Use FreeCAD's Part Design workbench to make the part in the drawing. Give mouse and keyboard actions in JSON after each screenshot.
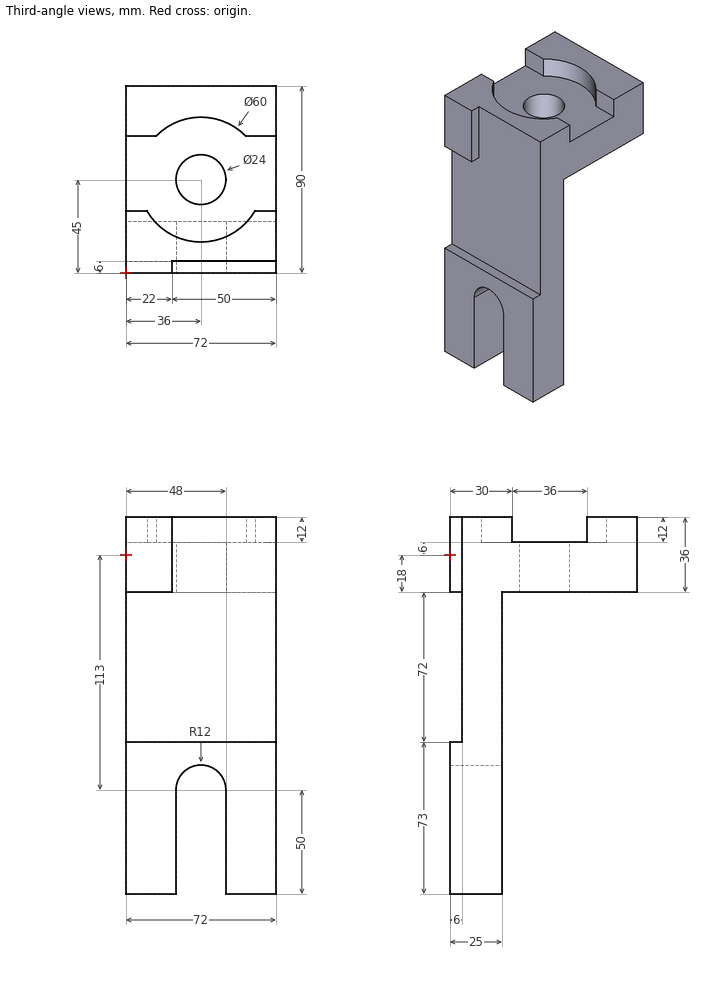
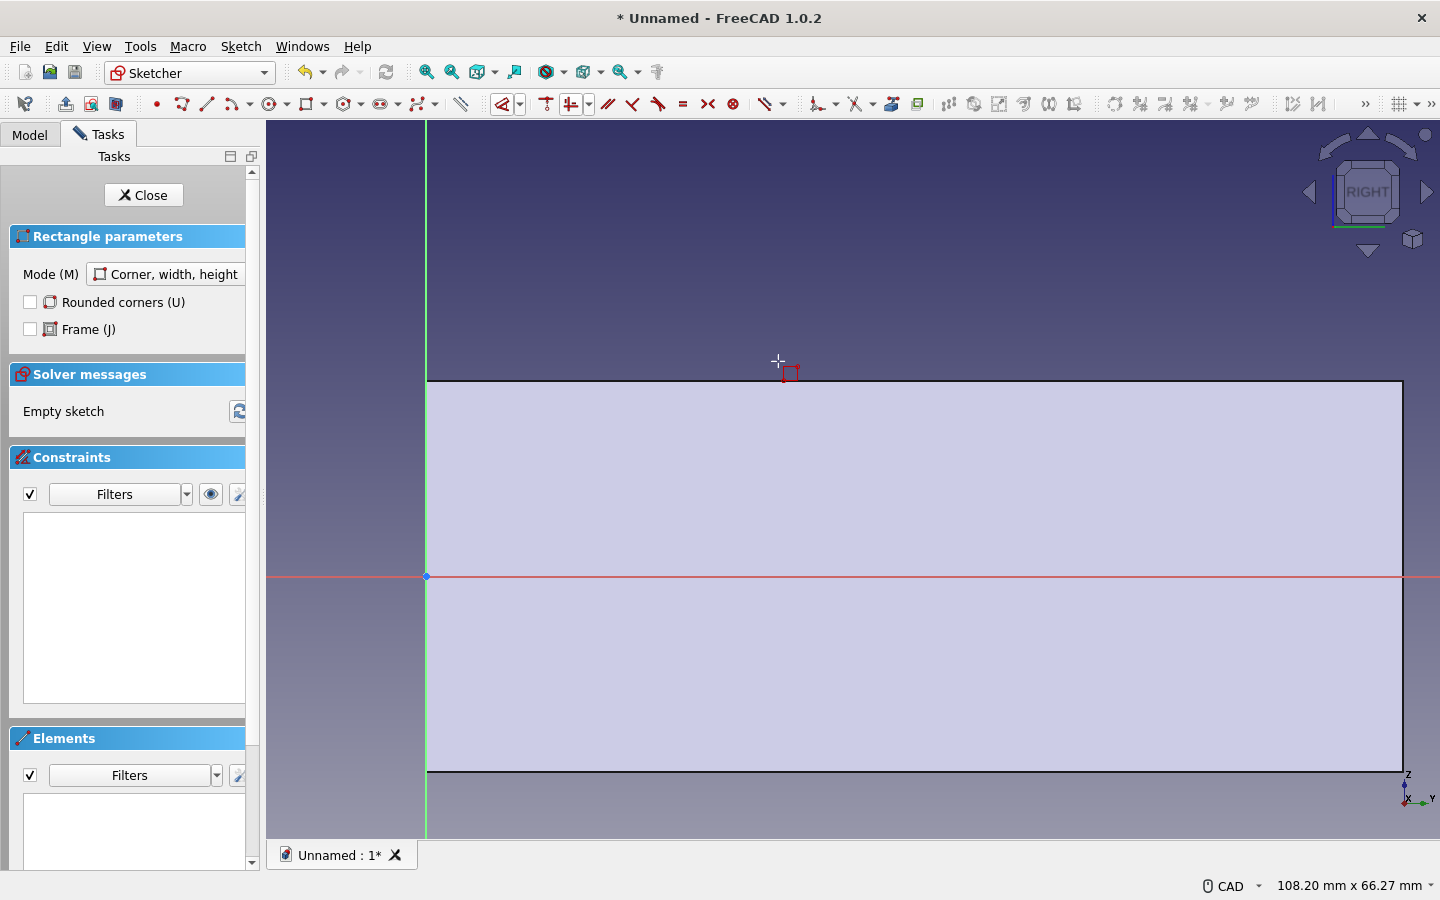
{"action": "left_click", "coordinate": [752, 381]}
{"action": "mouse_move", "coordinate": [1142, 512]}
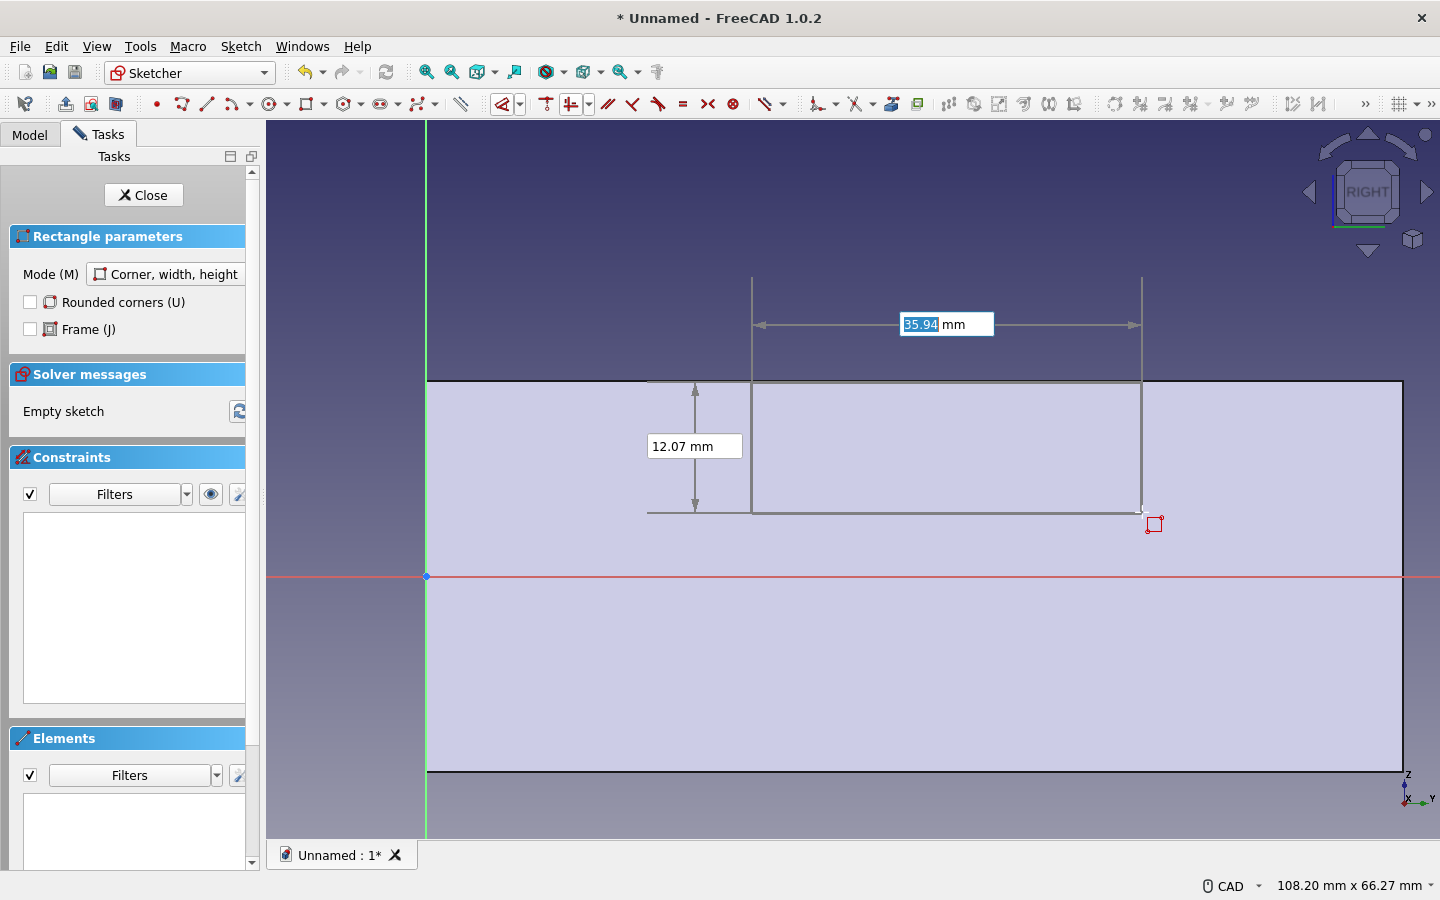
{"action": "type", "text": "36"}
{"action": "key", "text": "Tab"}
{"action": "type", "text": "12"}
{"action": "key", "text": "Return"}
{"action": "key", "text": "Escape"}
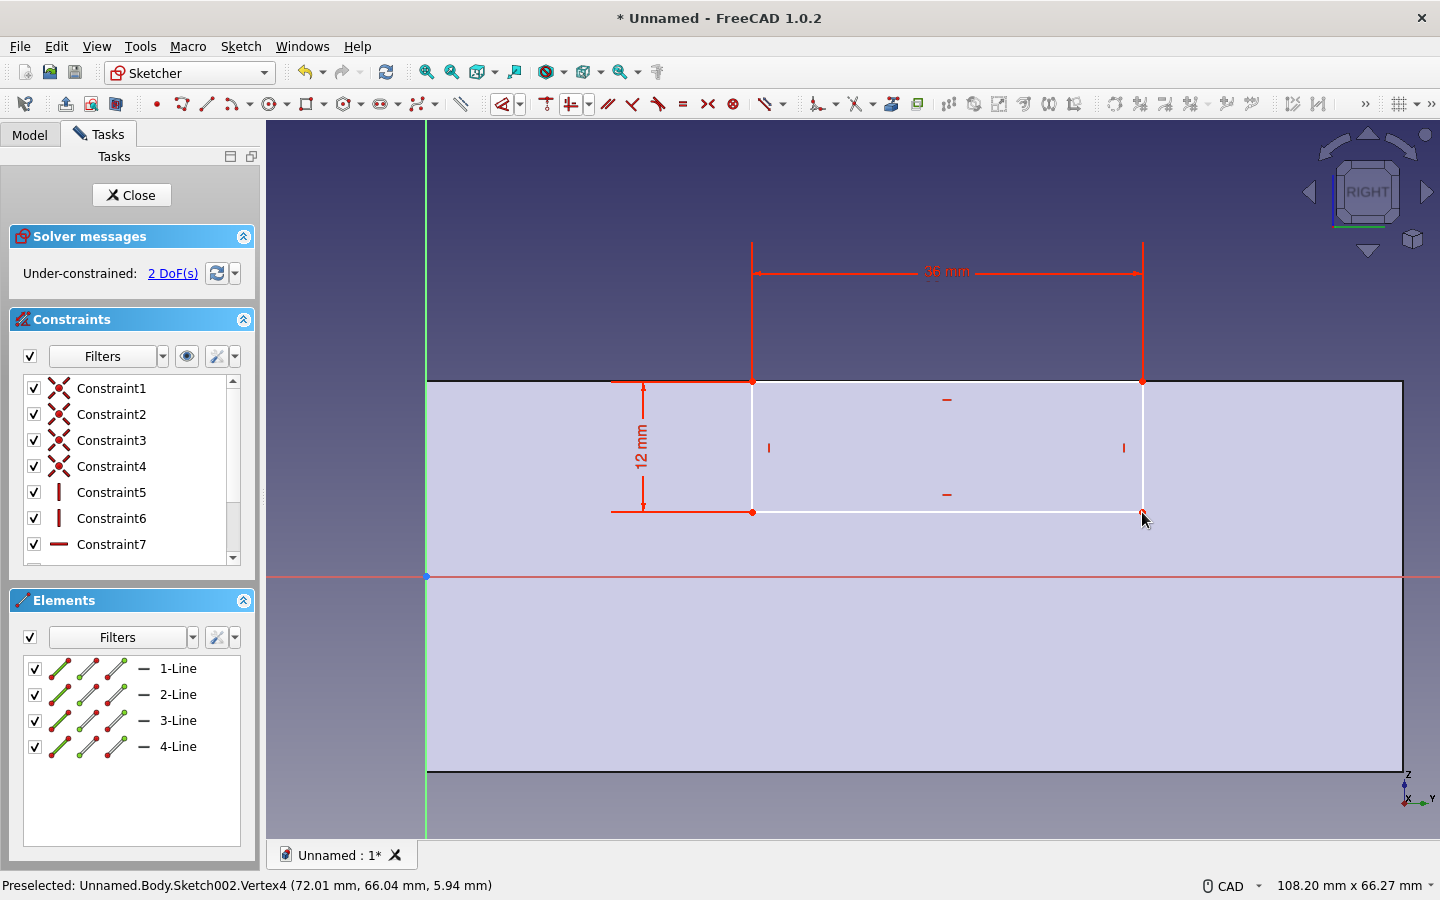
{"action": "key", "text": "d"}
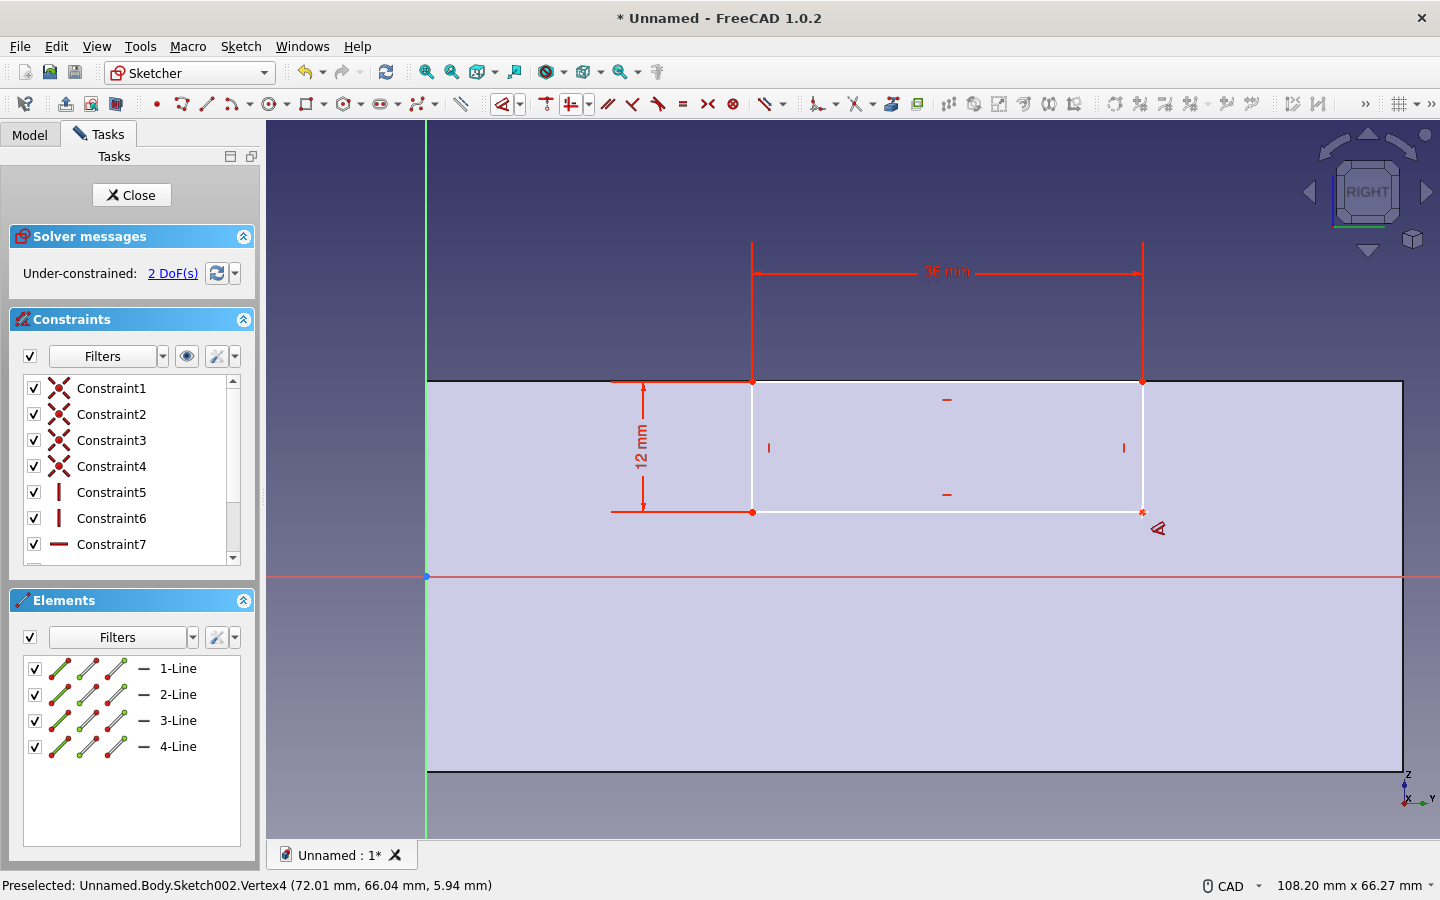
{"action": "left_click", "coordinate": [752, 512]}
{"action": "left_click", "coordinate": [392, 544]}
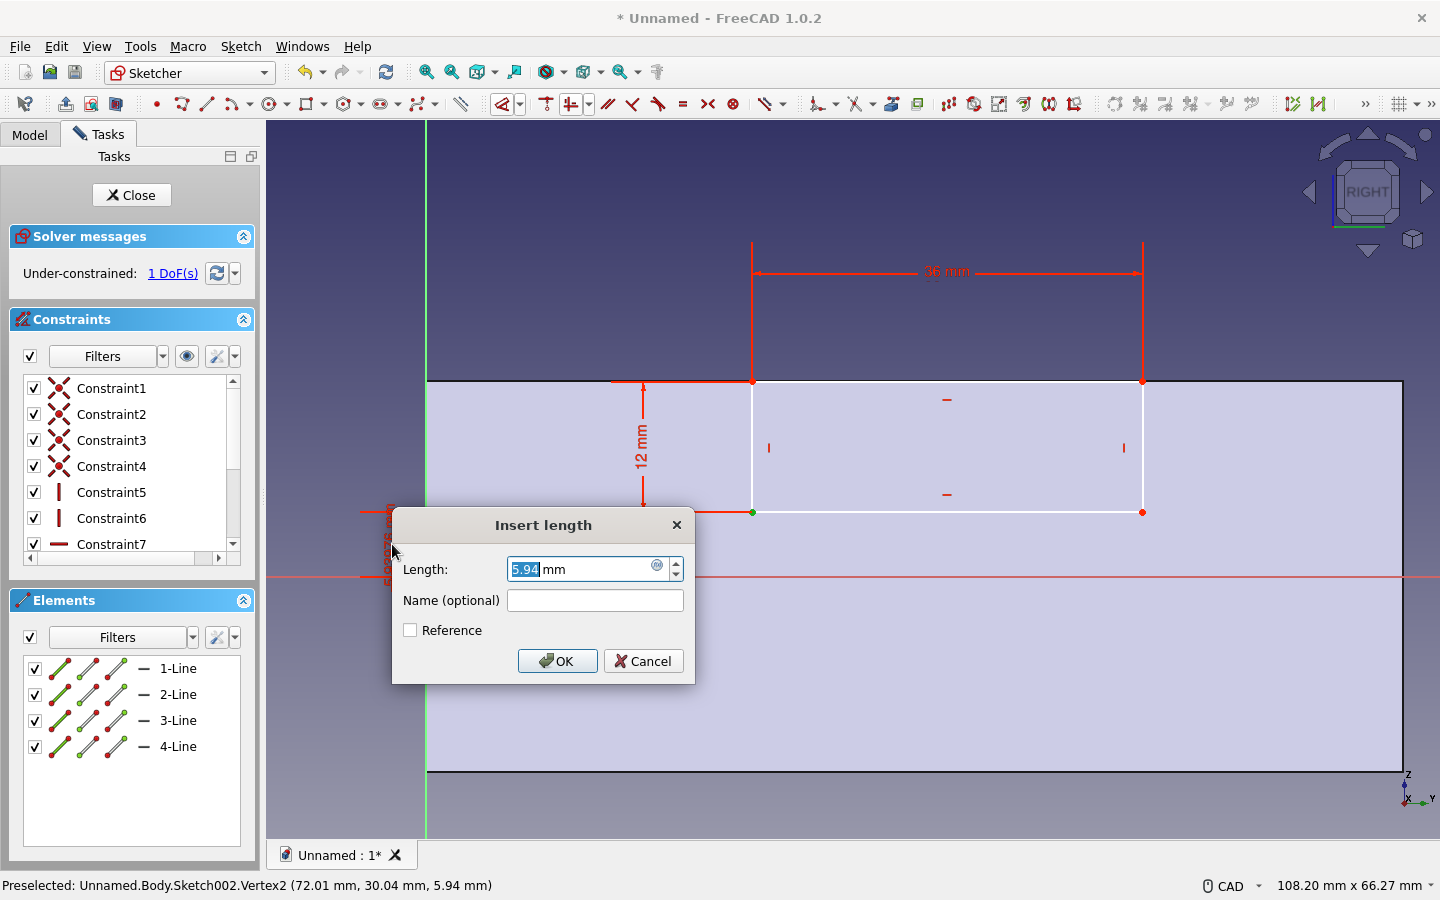
{"action": "type", "text": "6"}
{"action": "key", "text": "Return"}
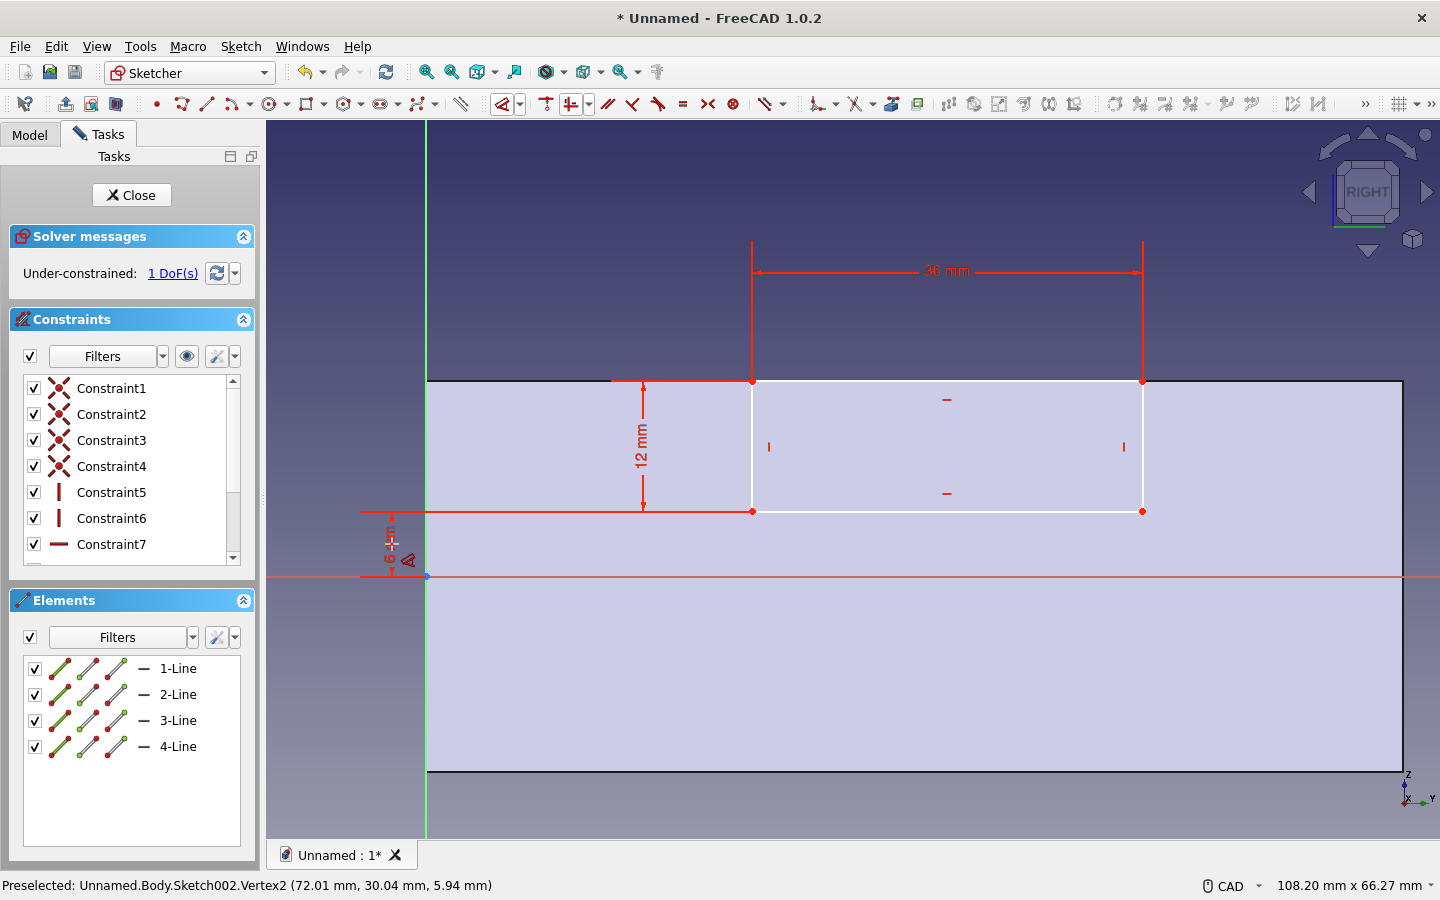
{"action": "left_click", "coordinate": [752, 381]}
{"action": "left_click", "coordinate": [589, 611]}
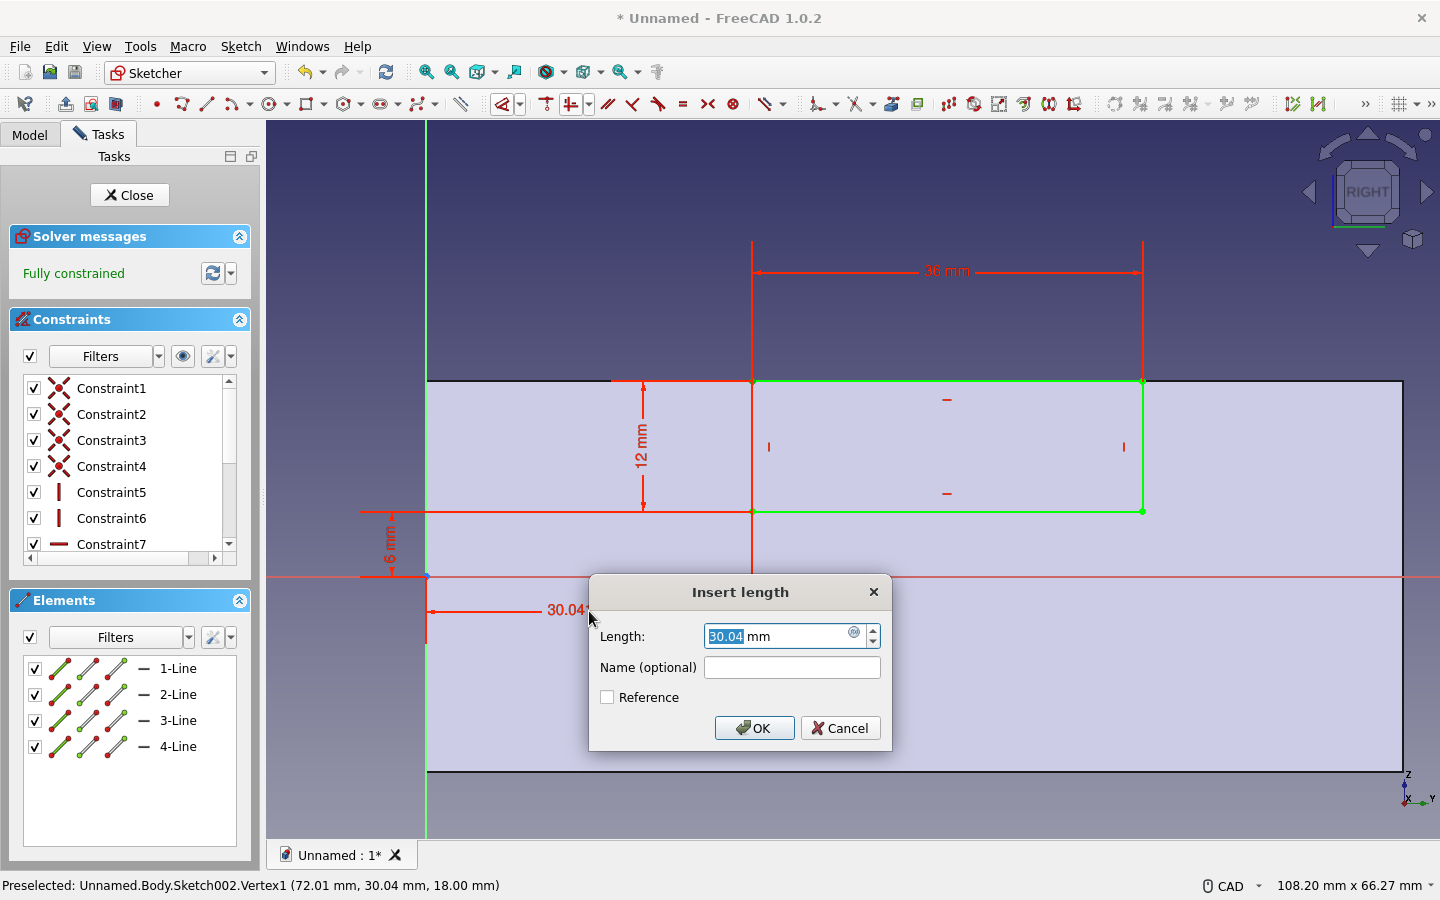
{"action": "type", "text": "30"}
{"action": "key", "text": "Return"}
{"action": "key", "text": "Escape"}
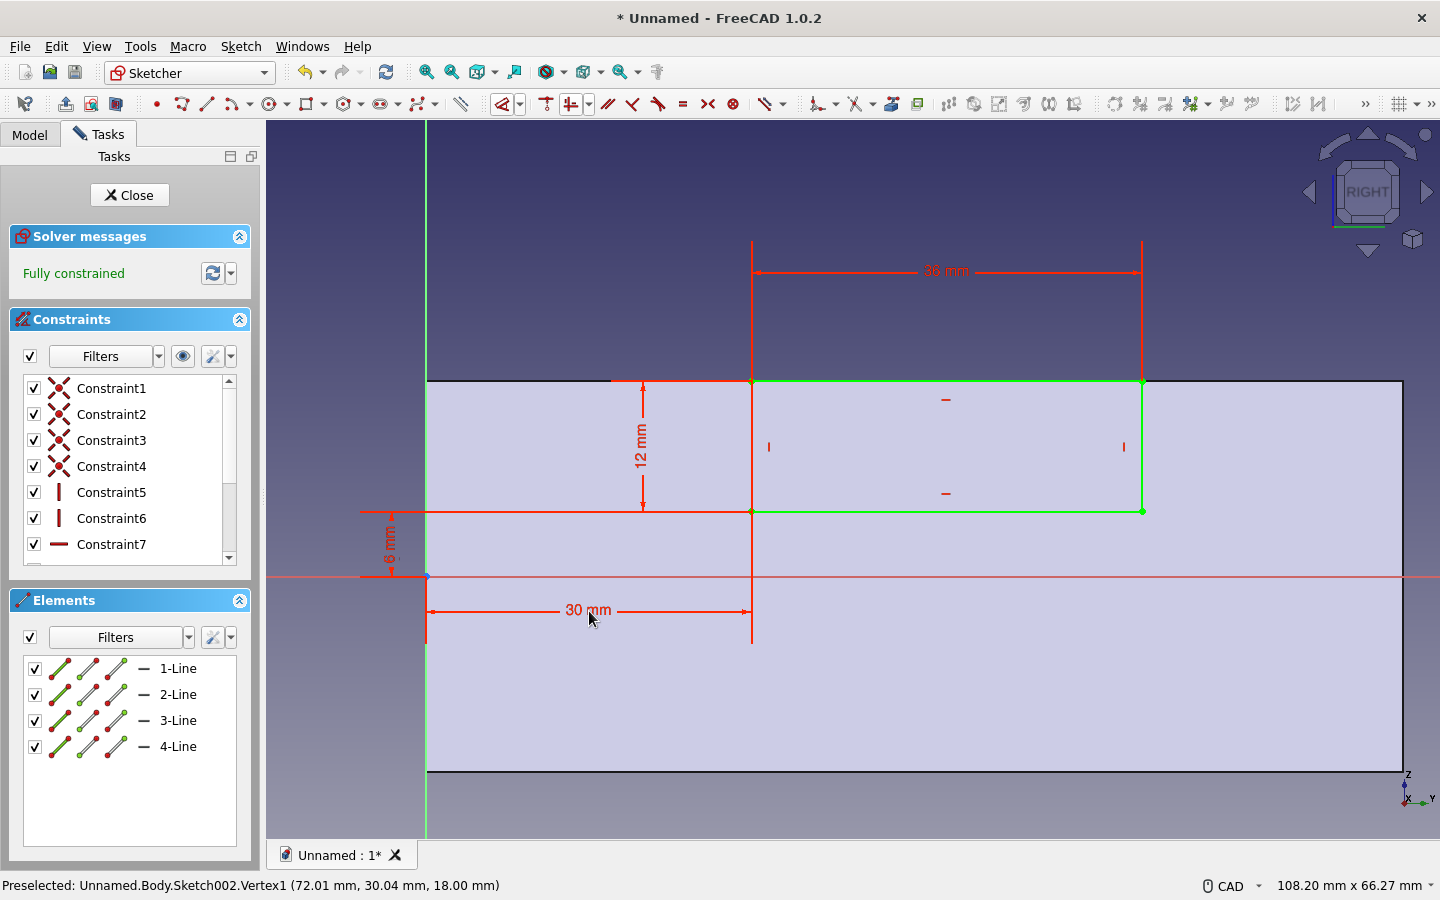
{"action": "left_click", "coordinate": [130, 195]}